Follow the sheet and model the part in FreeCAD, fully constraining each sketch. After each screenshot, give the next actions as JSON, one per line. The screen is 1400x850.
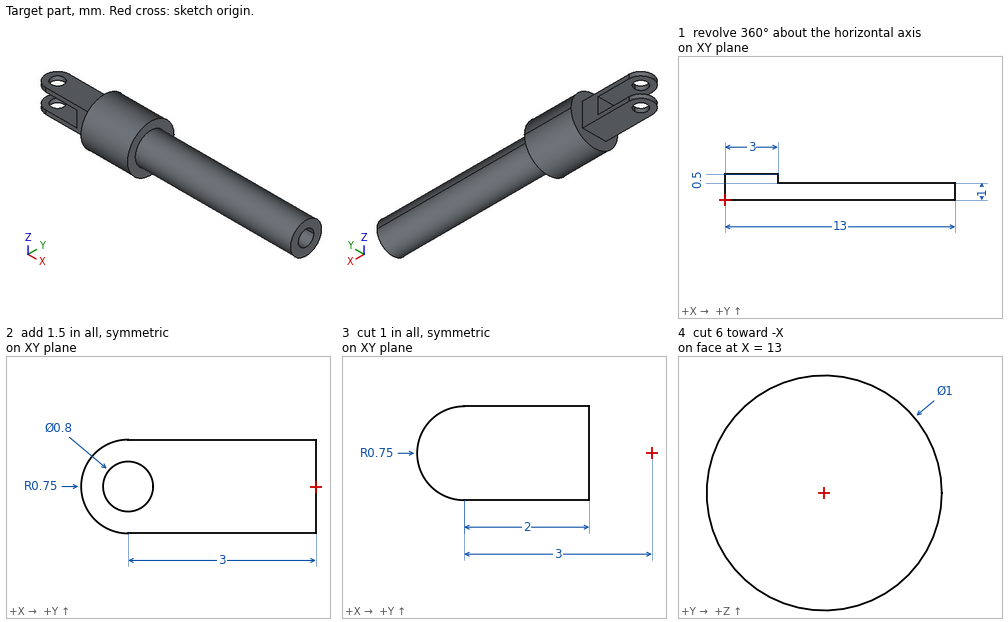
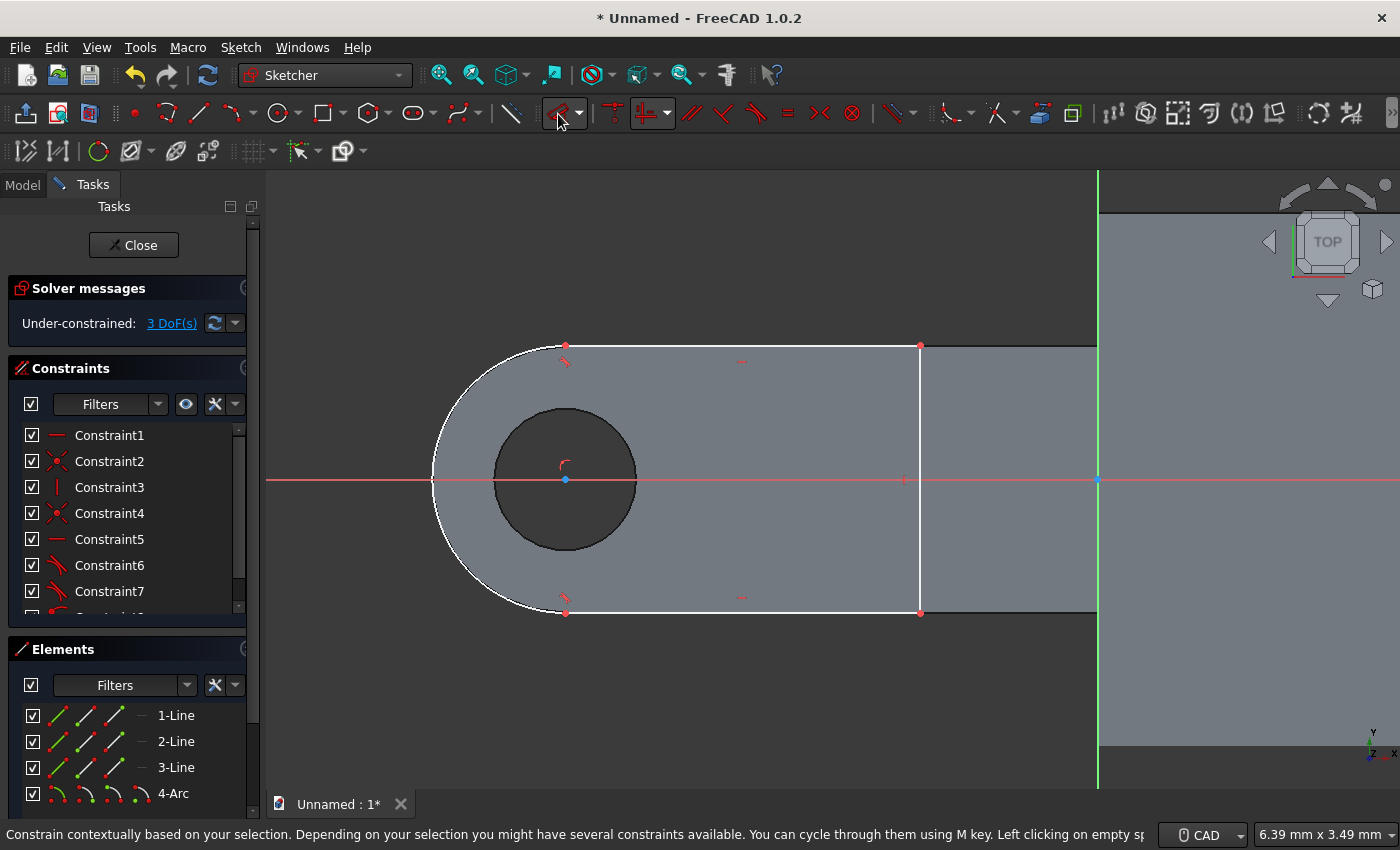
{"action": "left_click", "coordinate": [458, 401]}
{"action": "left_click", "coordinate": [432, 382]}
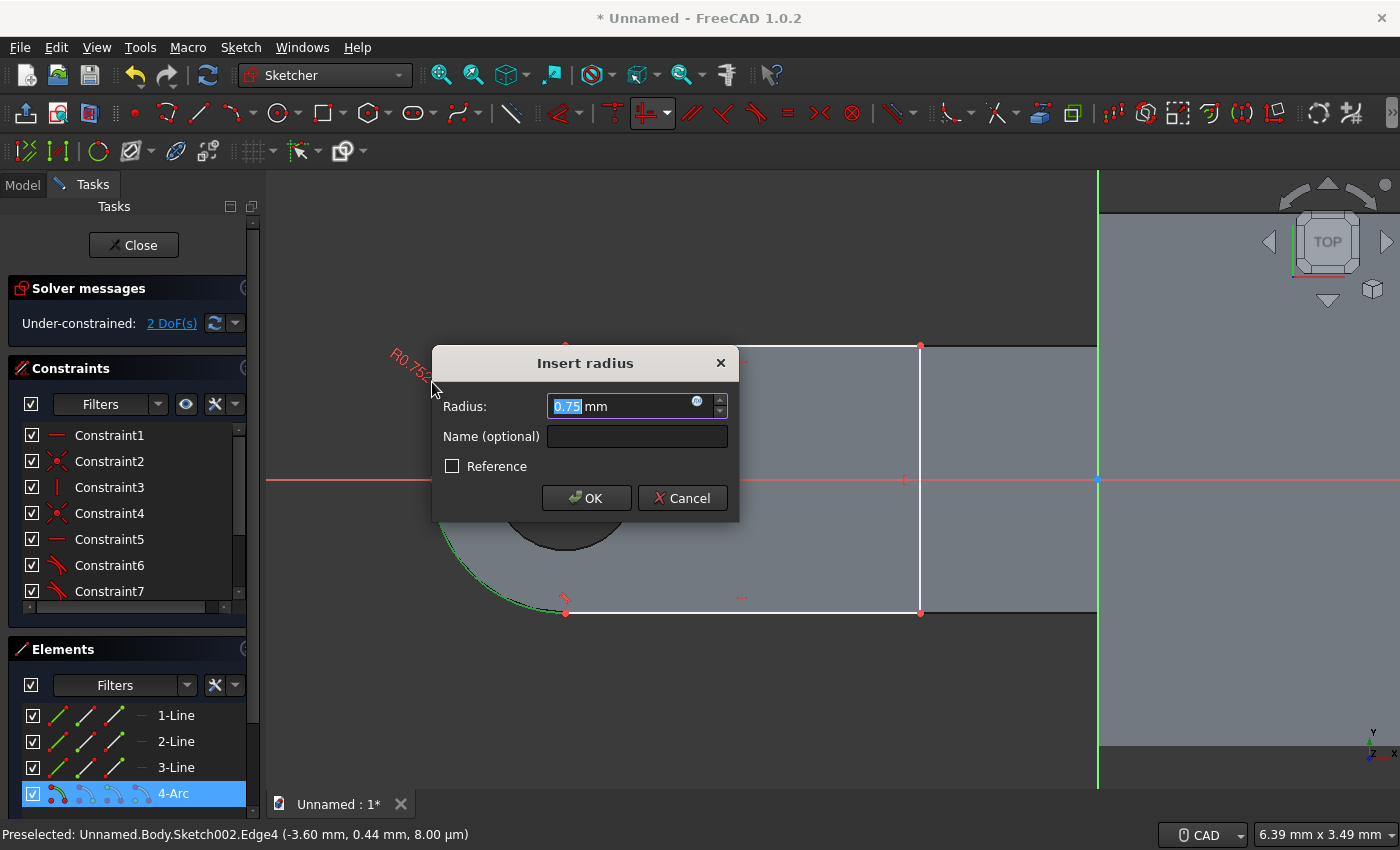
{"action": "type", "text": "0.75"}
{"action": "key", "text": "Return"}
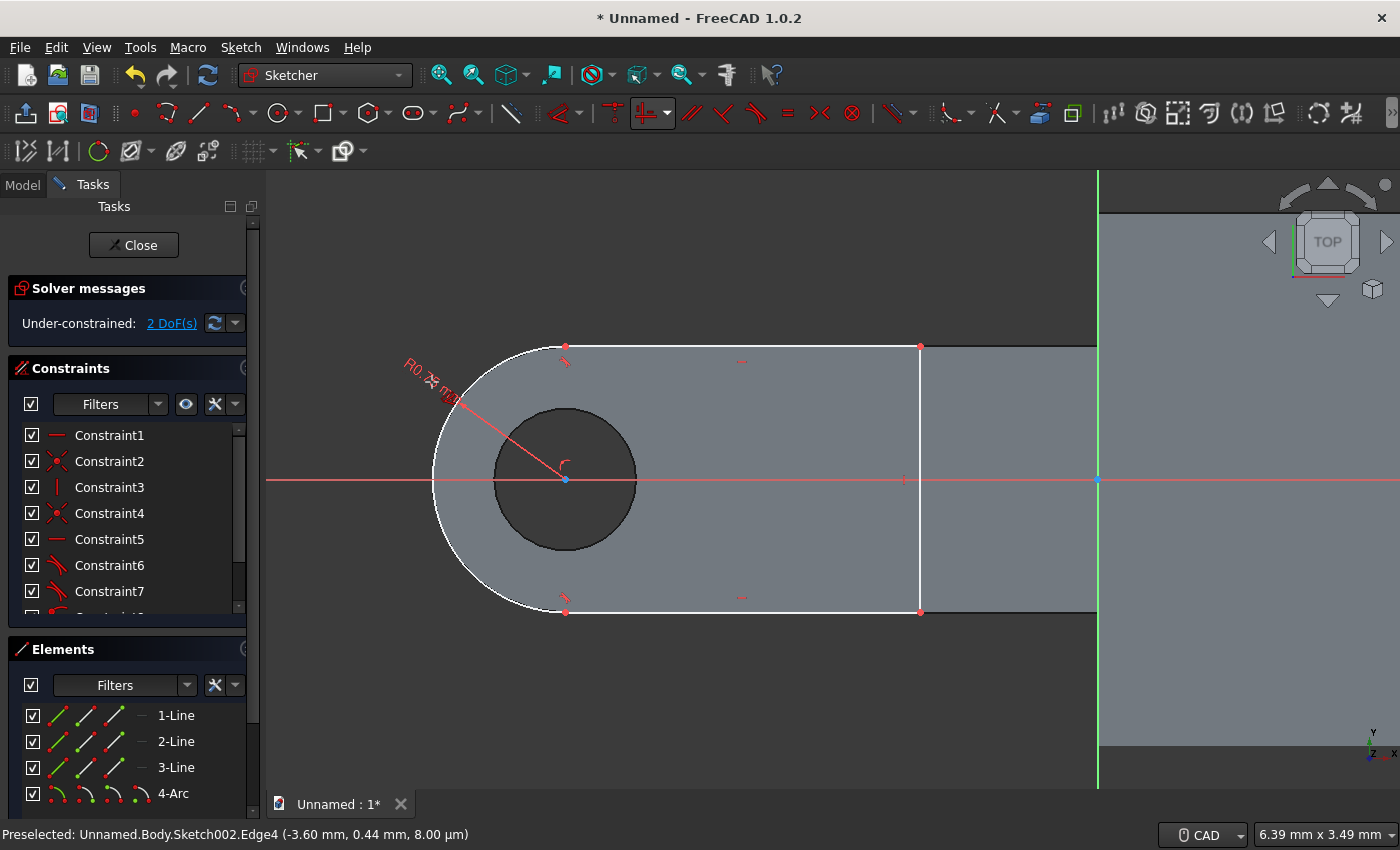
{"action": "left_click", "coordinate": [672, 613]}
{"action": "left_click", "coordinate": [743, 647]}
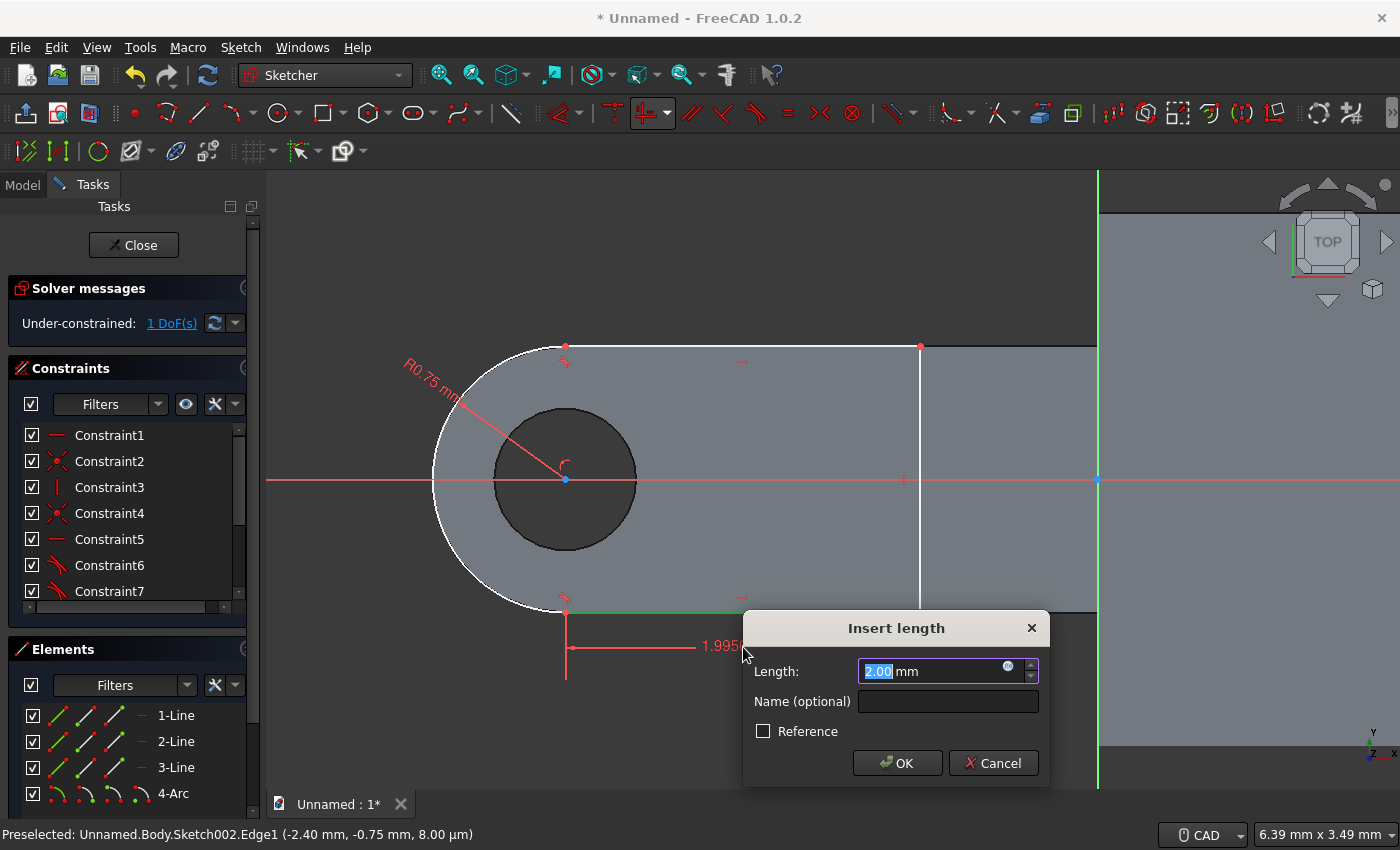
{"action": "type", "text": "2"}
{"action": "key", "text": "Return"}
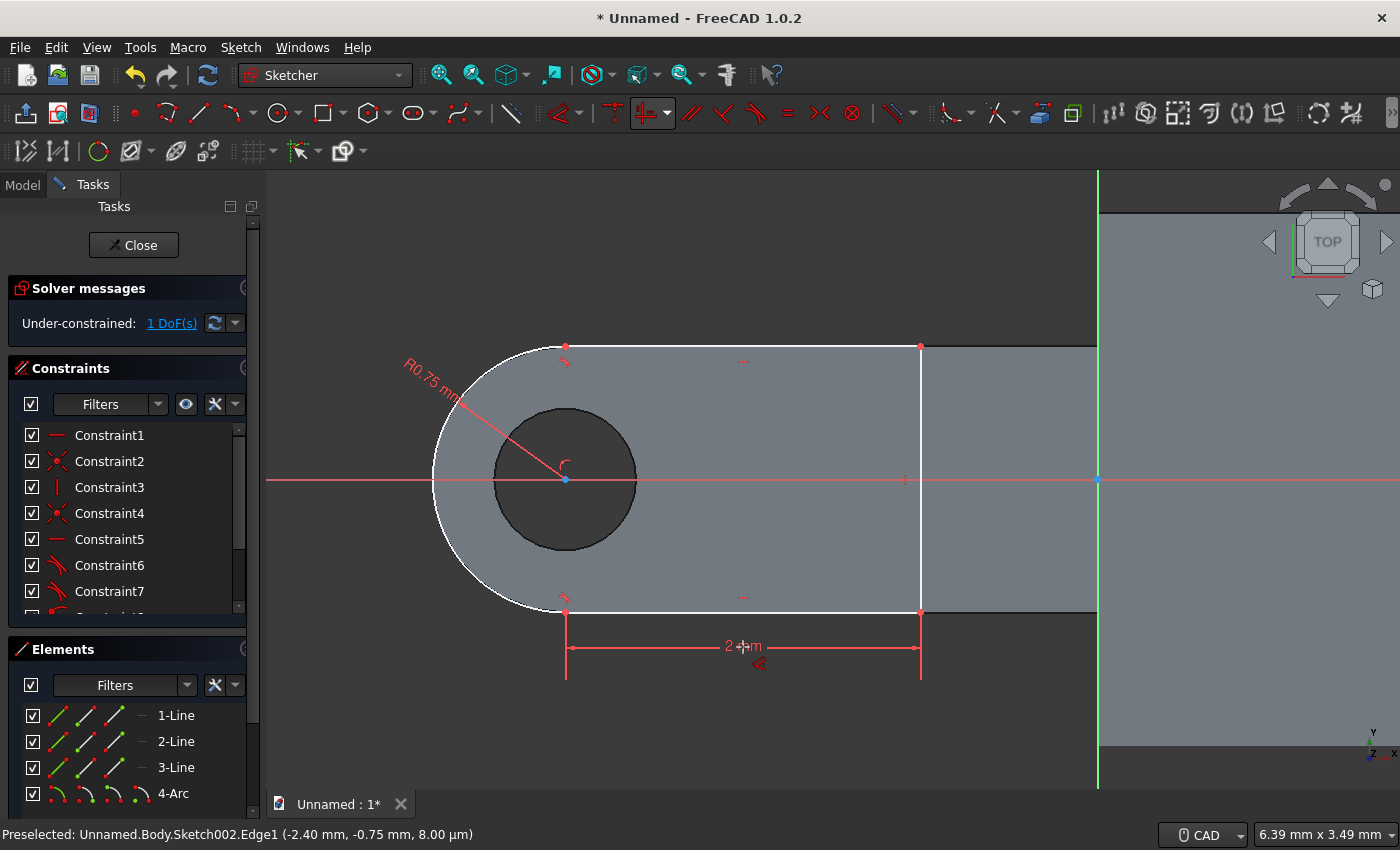
{"action": "left_click", "coordinate": [566, 613]}
{"action": "left_click", "coordinate": [832, 647]}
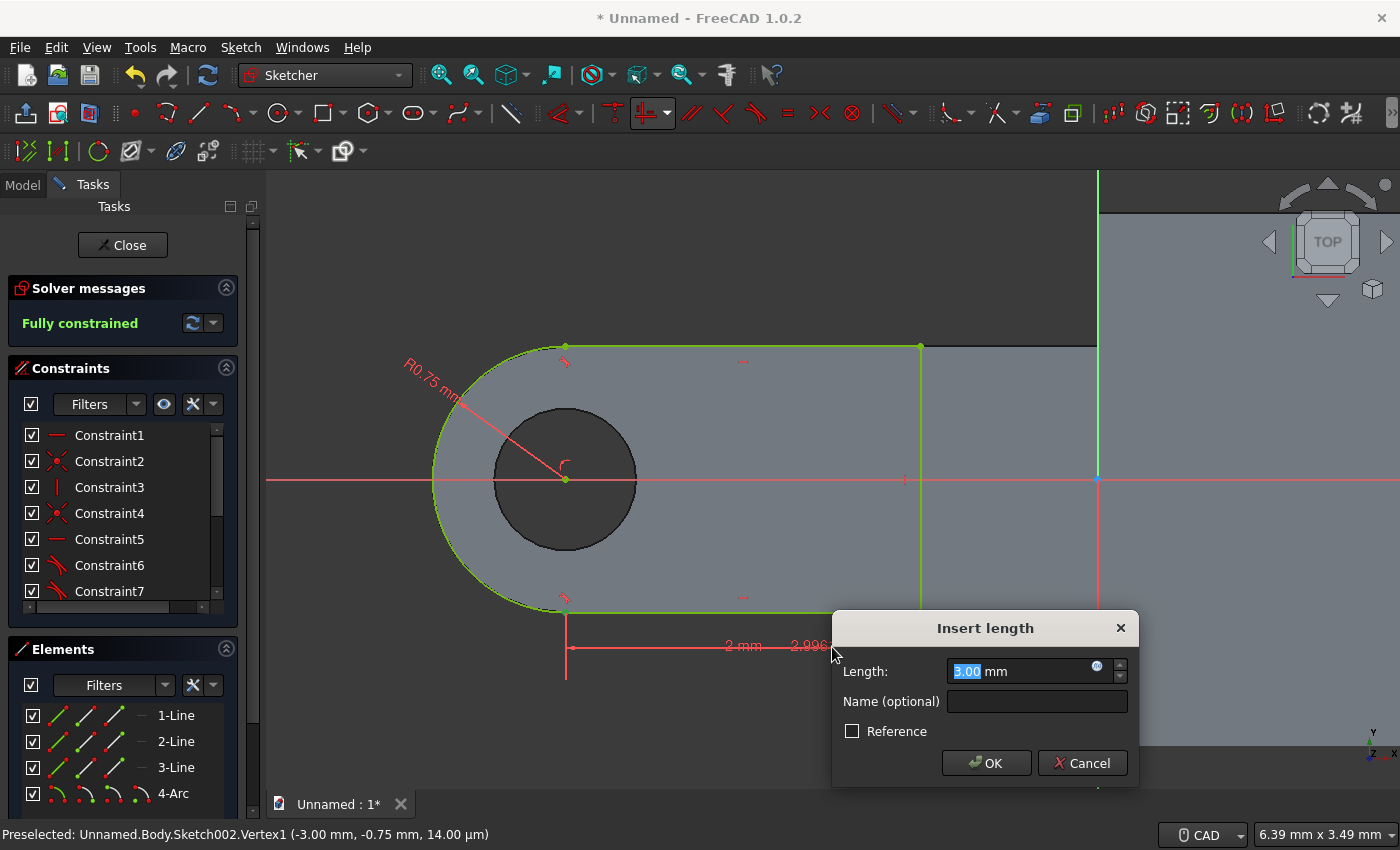
{"action": "type", "text": "3"}
{"action": "key", "text": "Return"}
{"action": "key", "text": "Escape"}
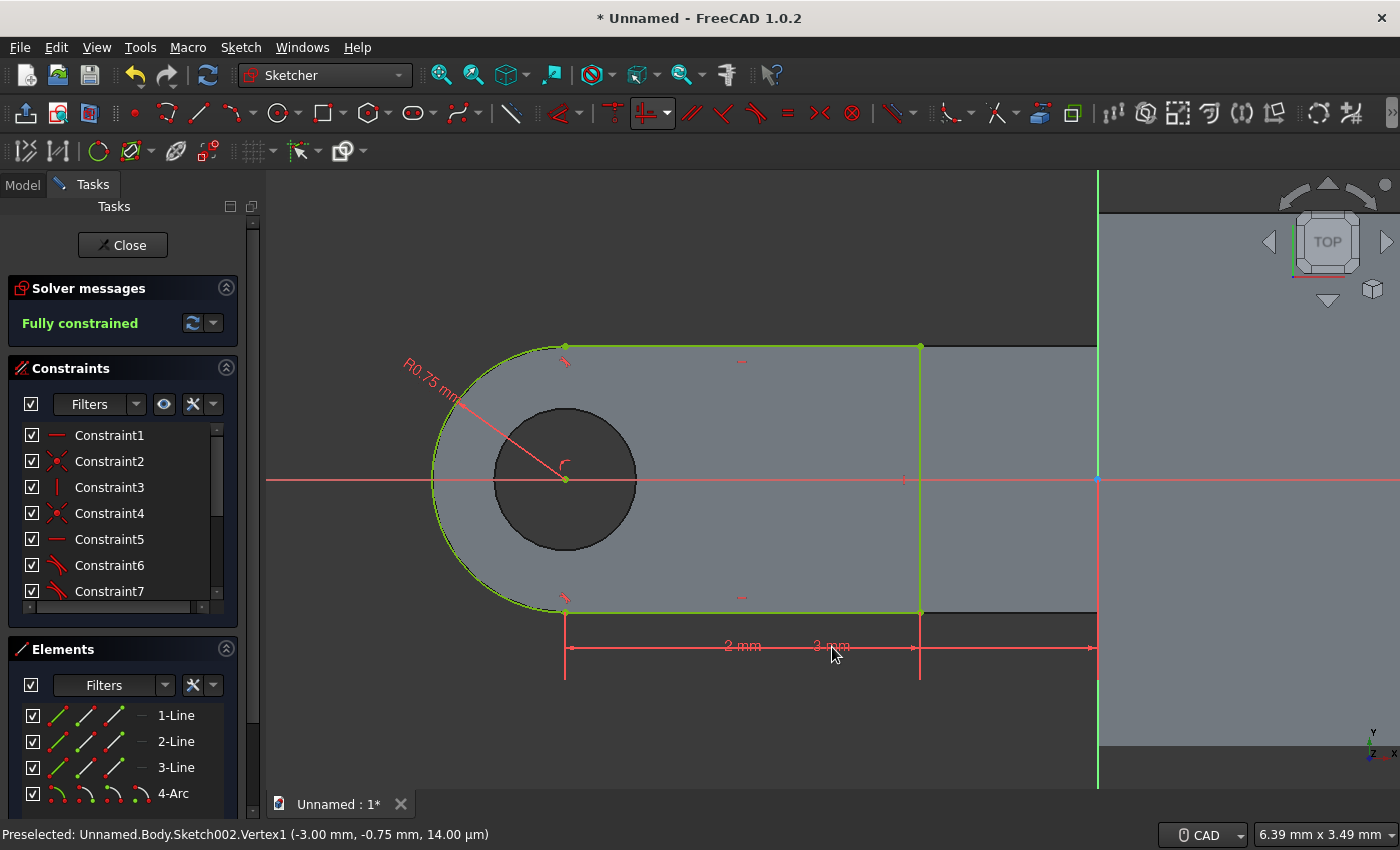
{"action": "left_click", "coordinate": [123, 245]}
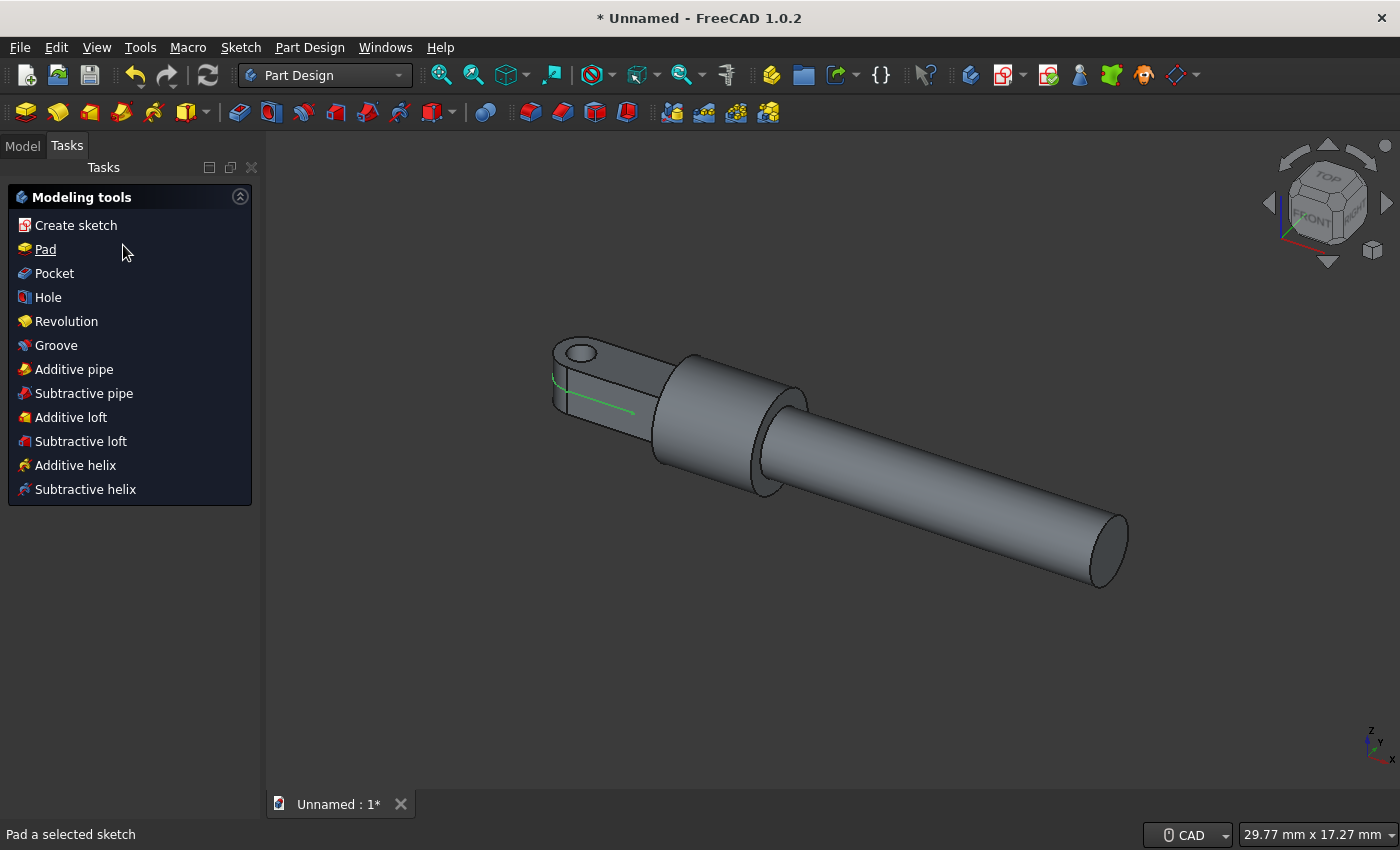
{"action": "left_click", "coordinate": [240, 112]}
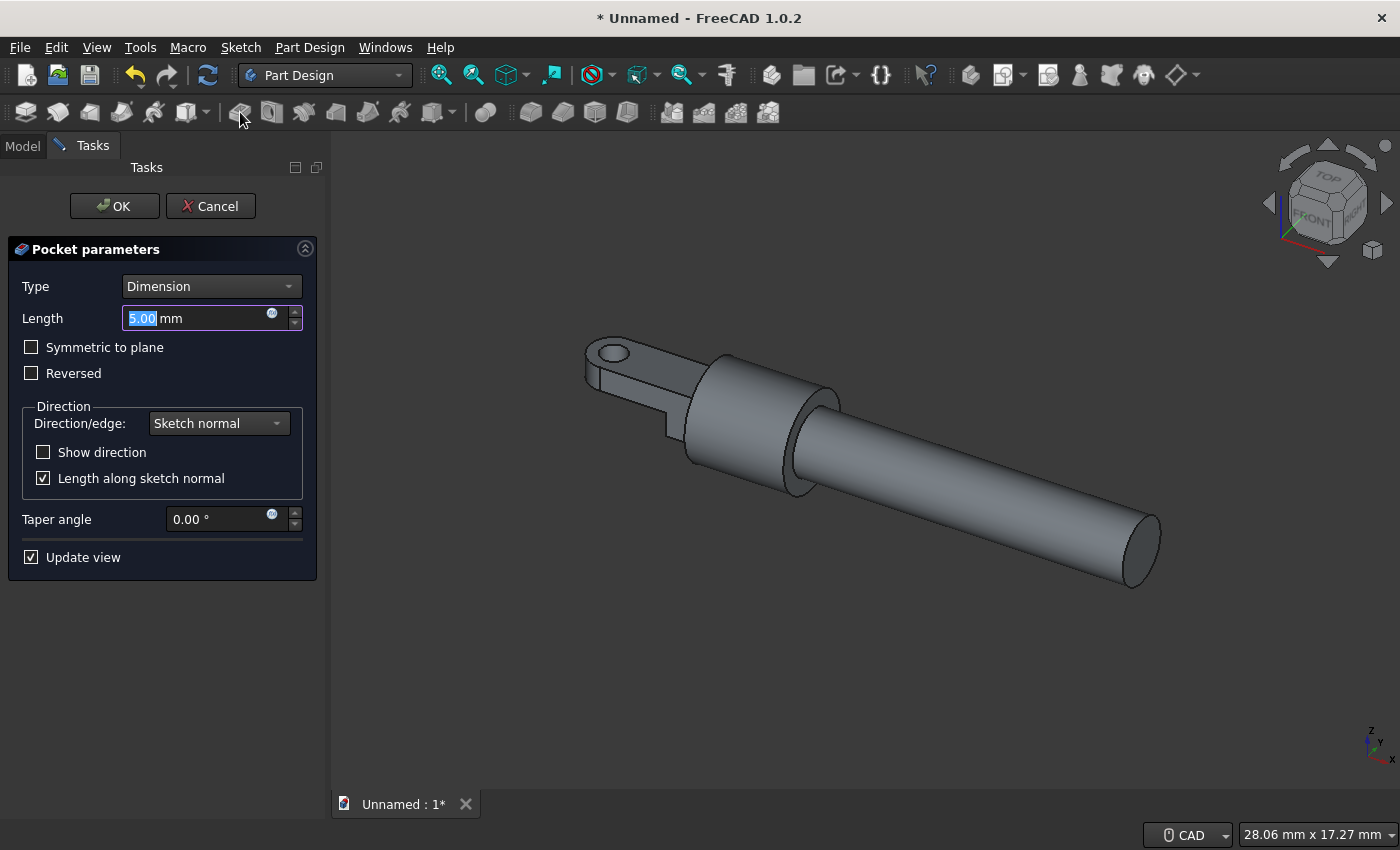
{"action": "type", "text": "1"}
{"action": "key", "text": "Tab"}